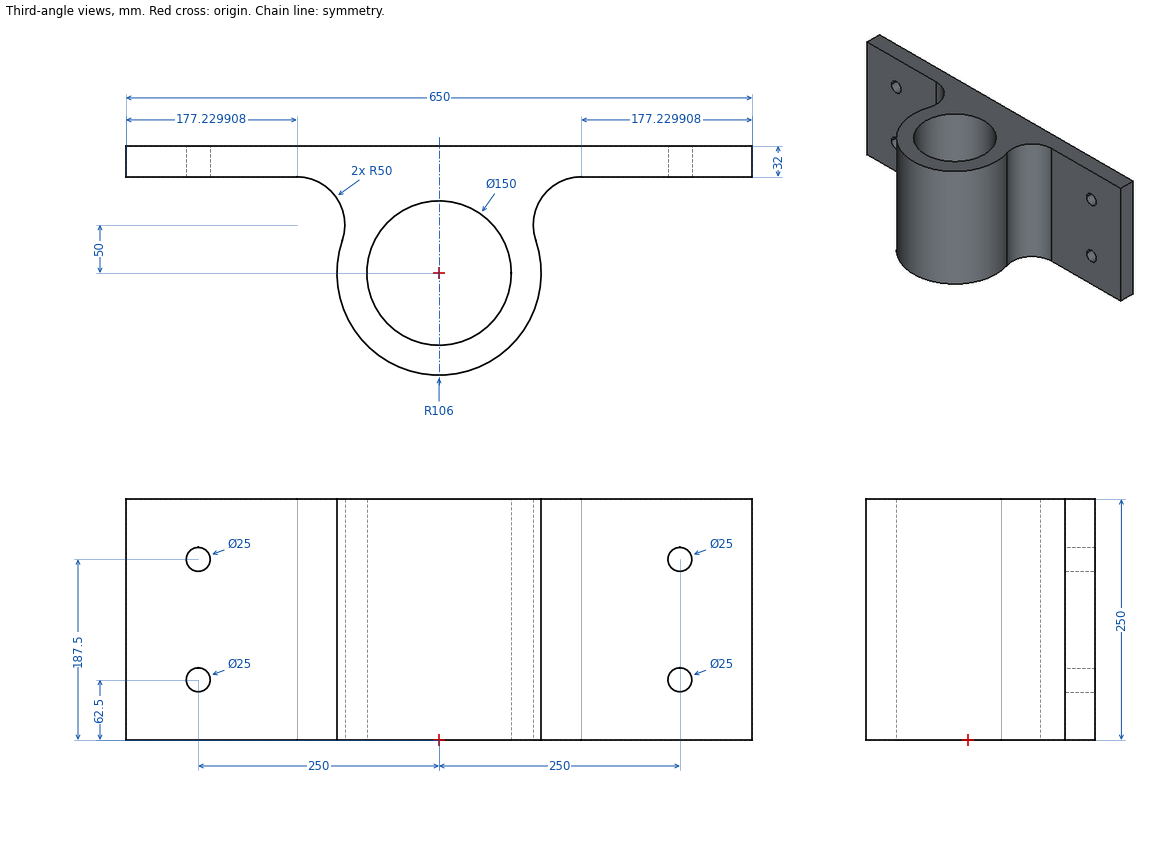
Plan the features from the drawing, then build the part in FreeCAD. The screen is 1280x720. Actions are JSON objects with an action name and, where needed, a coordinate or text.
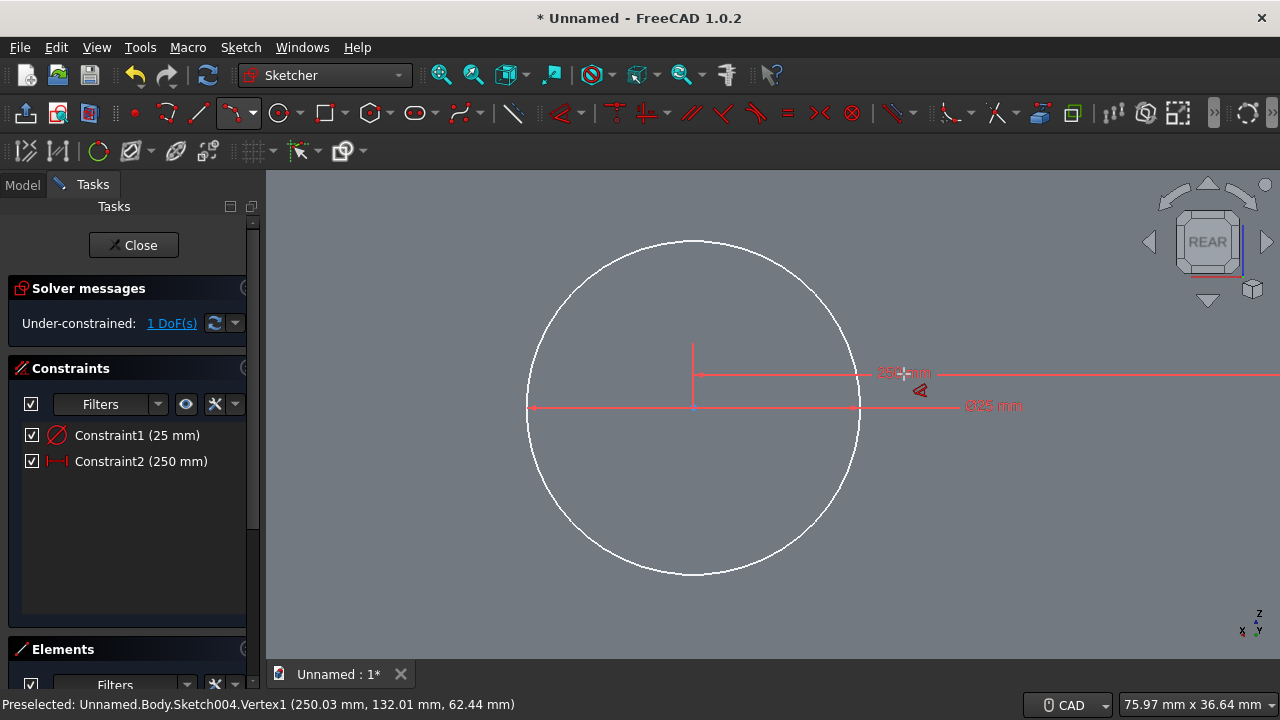
{"action": "left_click", "coordinate": [693, 408]}
{"action": "left_click", "coordinate": [659, 520]}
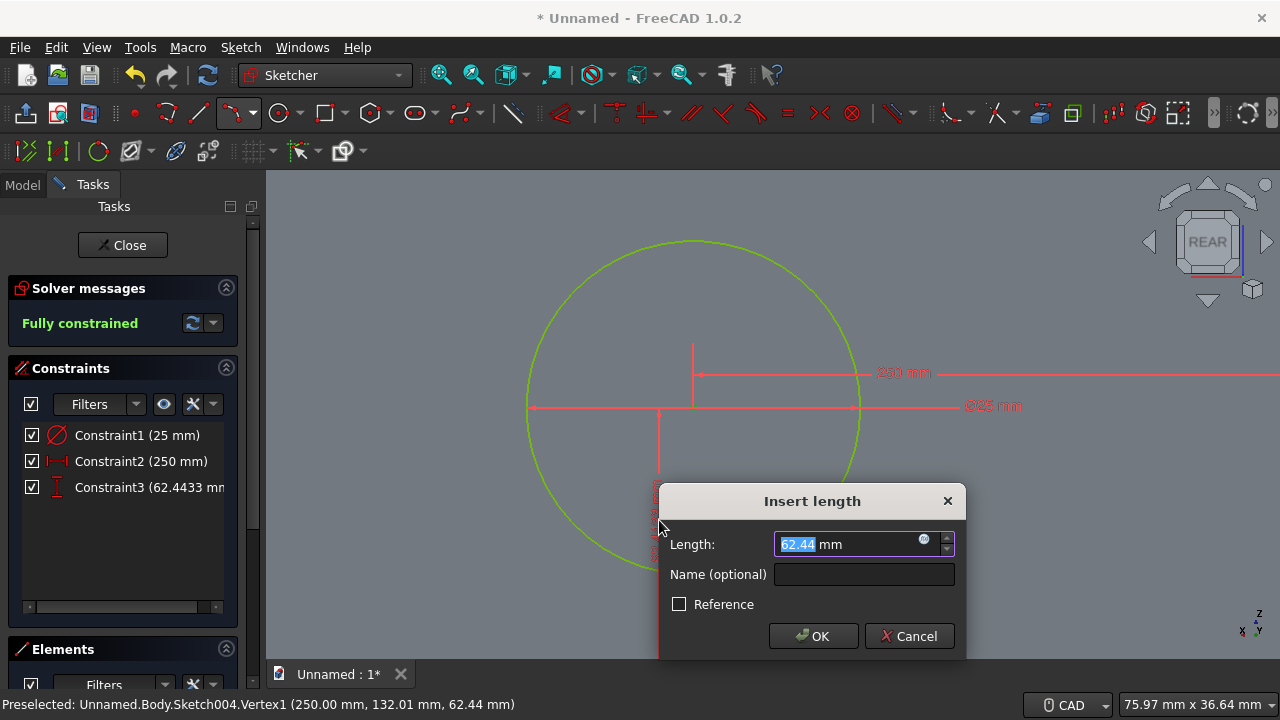
{"action": "type", "text": "62.5"}
{"action": "key", "text": "Return"}
{"action": "key", "text": "Escape"}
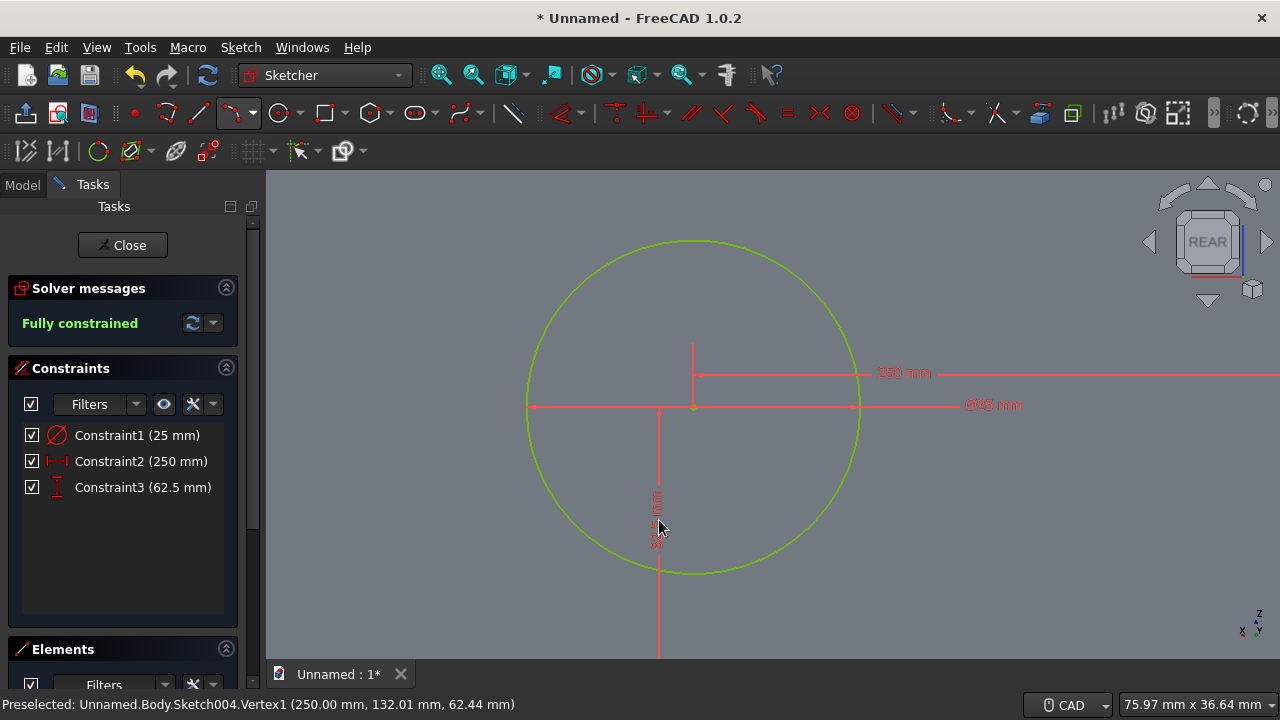
{"action": "left_click", "coordinate": [123, 245]}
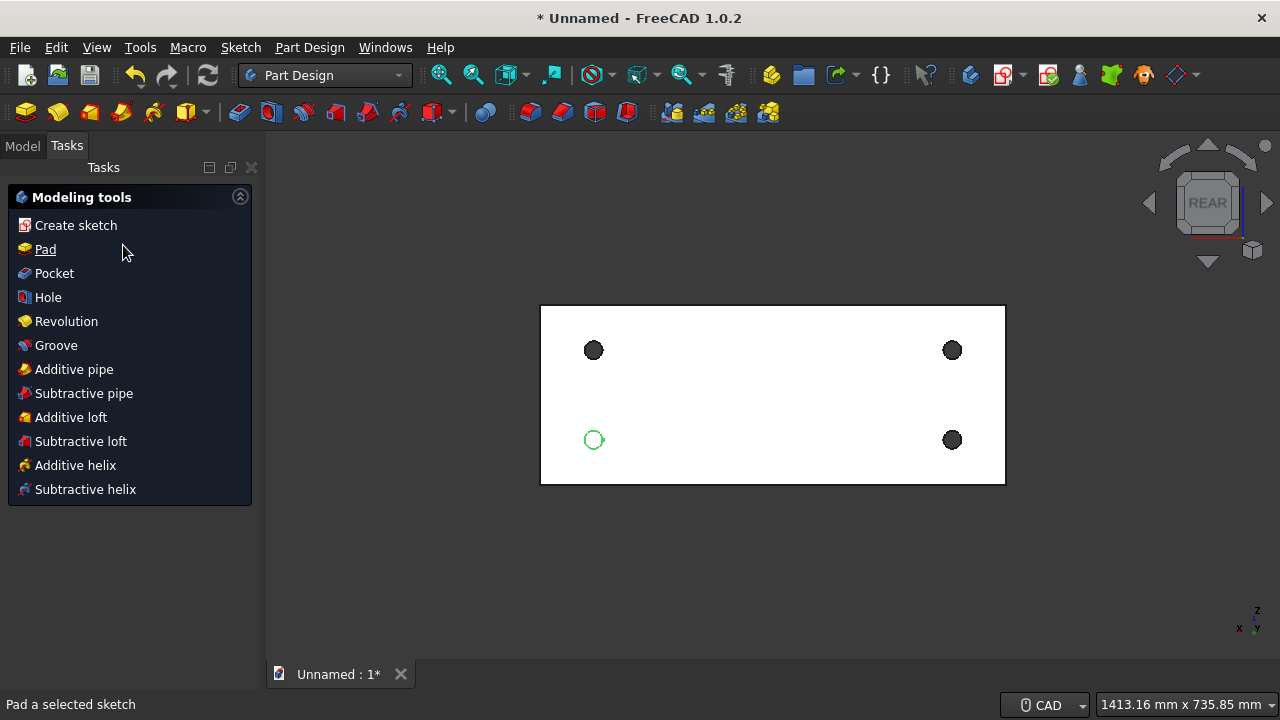
{"action": "left_click", "coordinate": [240, 112]}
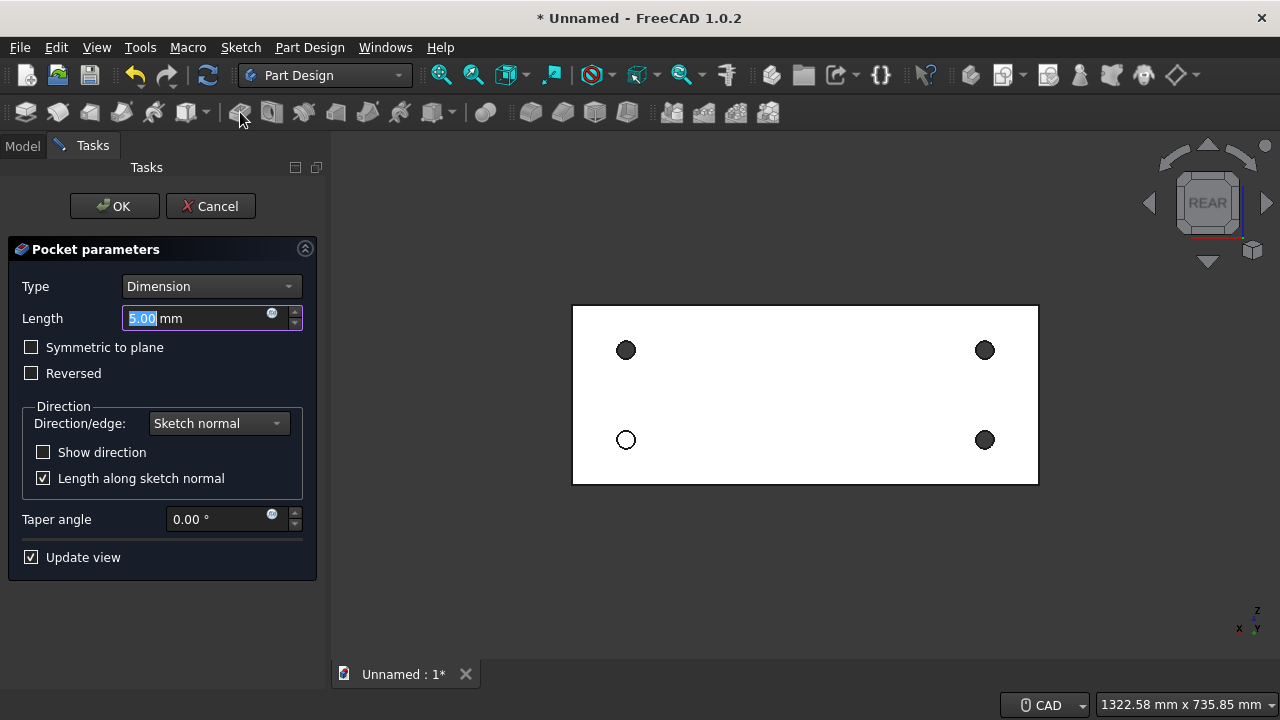
{"action": "left_click", "coordinate": [212, 286]}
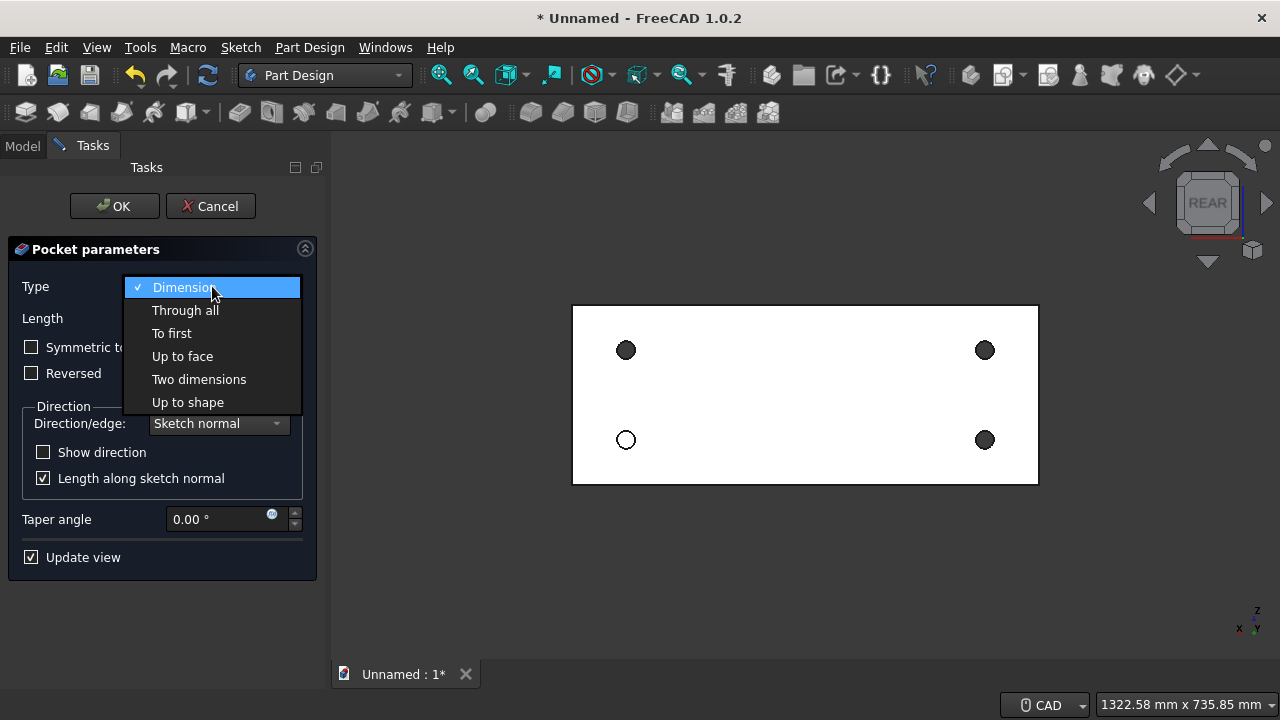
{"action": "left_click", "coordinate": [212, 334]}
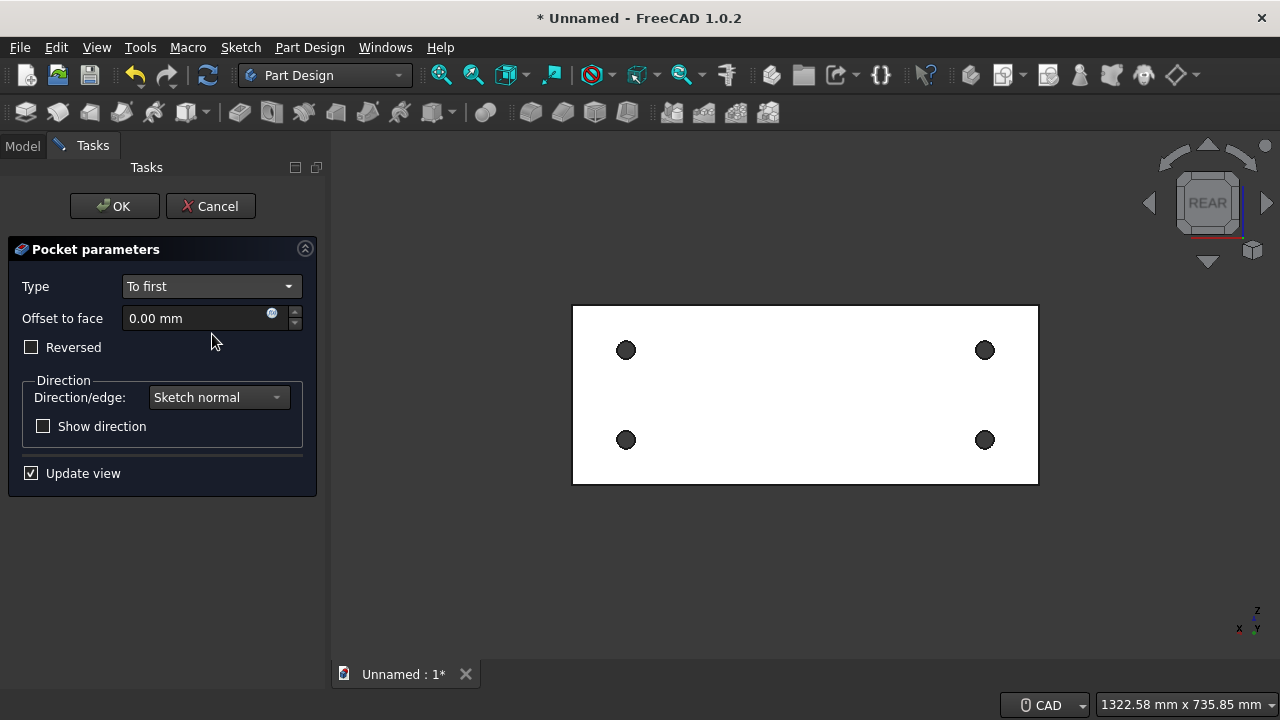
{"action": "left_click", "coordinate": [115, 206]}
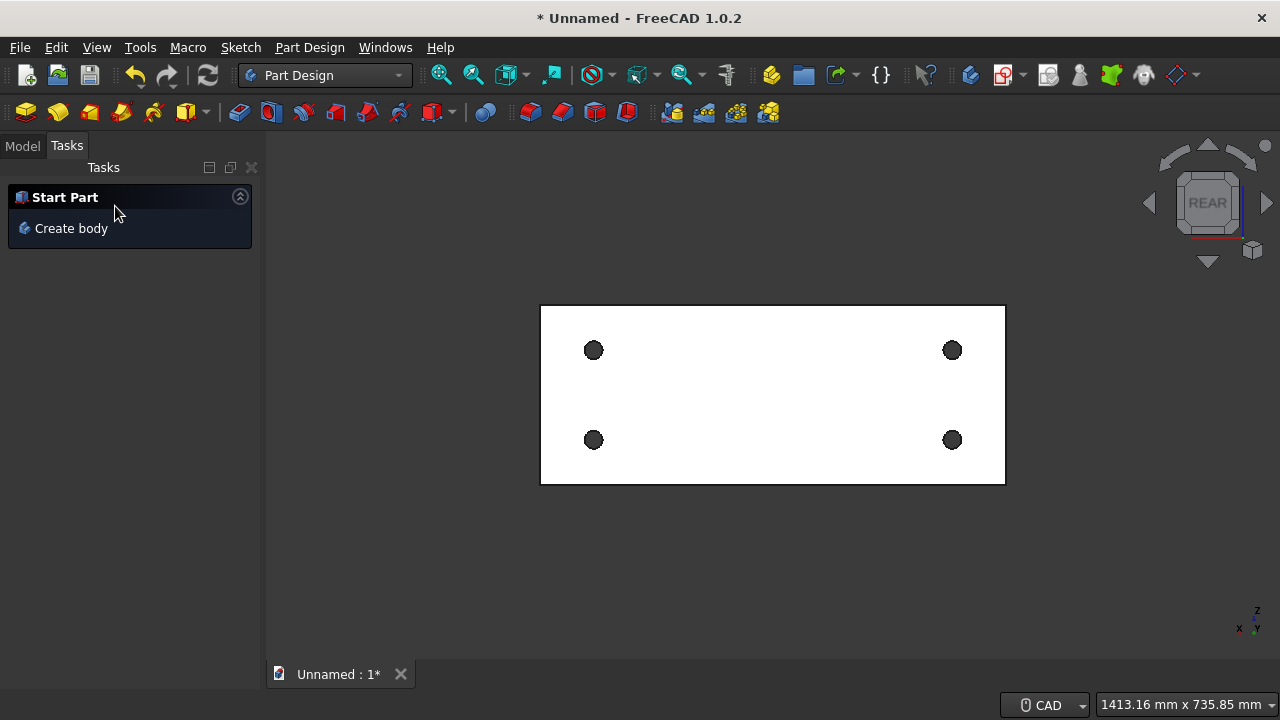
{"action": "key", "text": "0"}